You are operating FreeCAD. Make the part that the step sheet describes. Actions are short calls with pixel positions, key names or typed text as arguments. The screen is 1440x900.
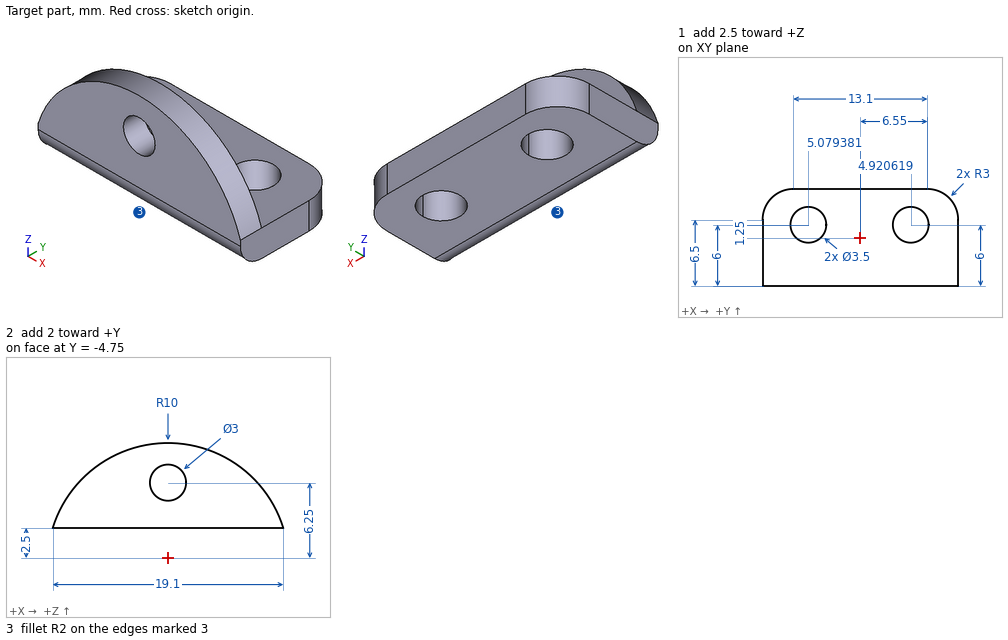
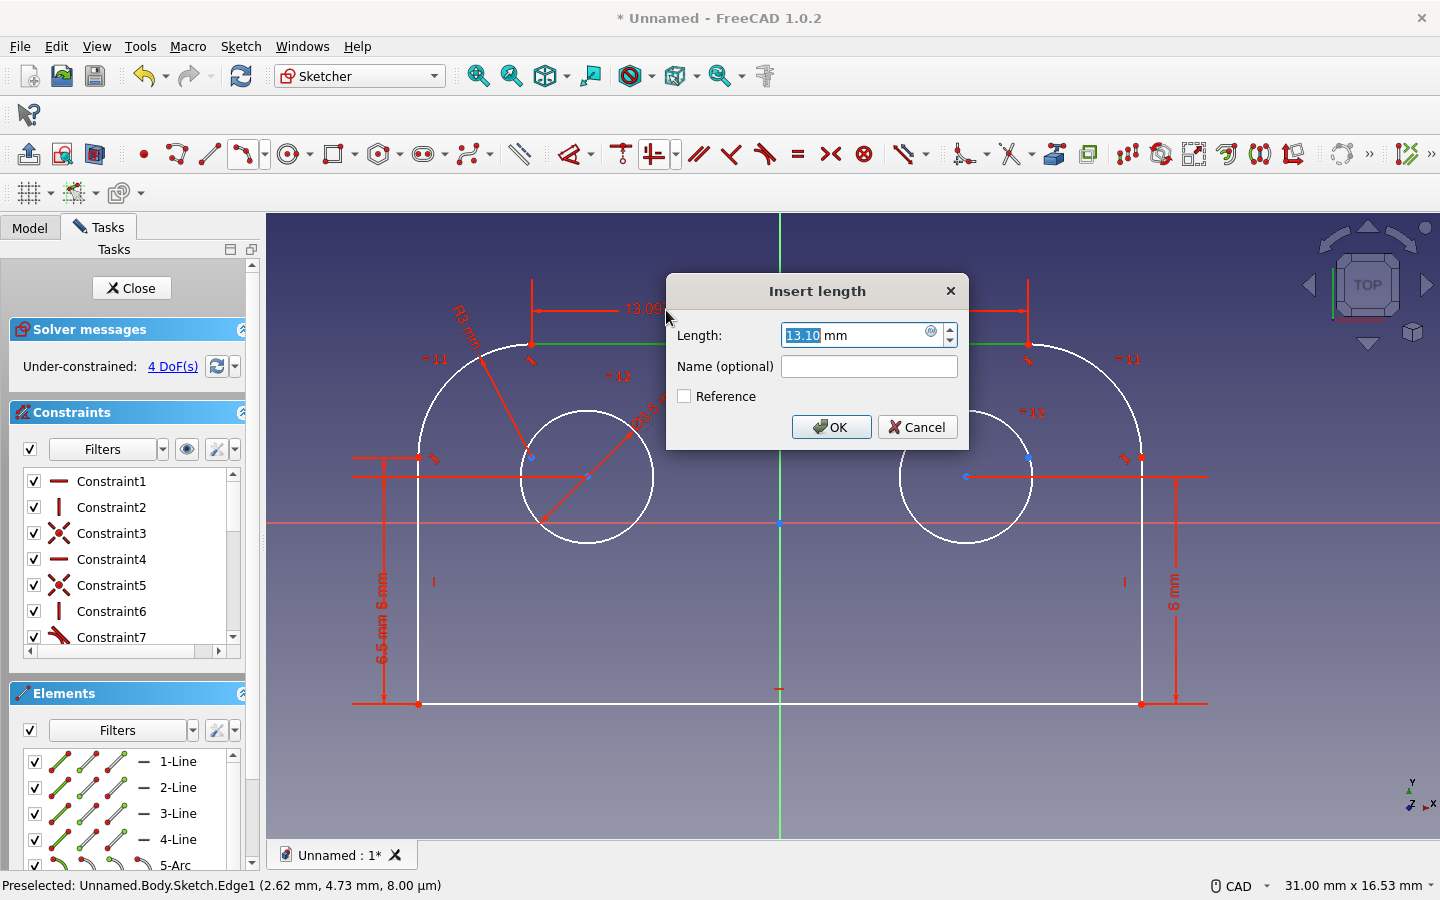
text(13.1)
key(Return)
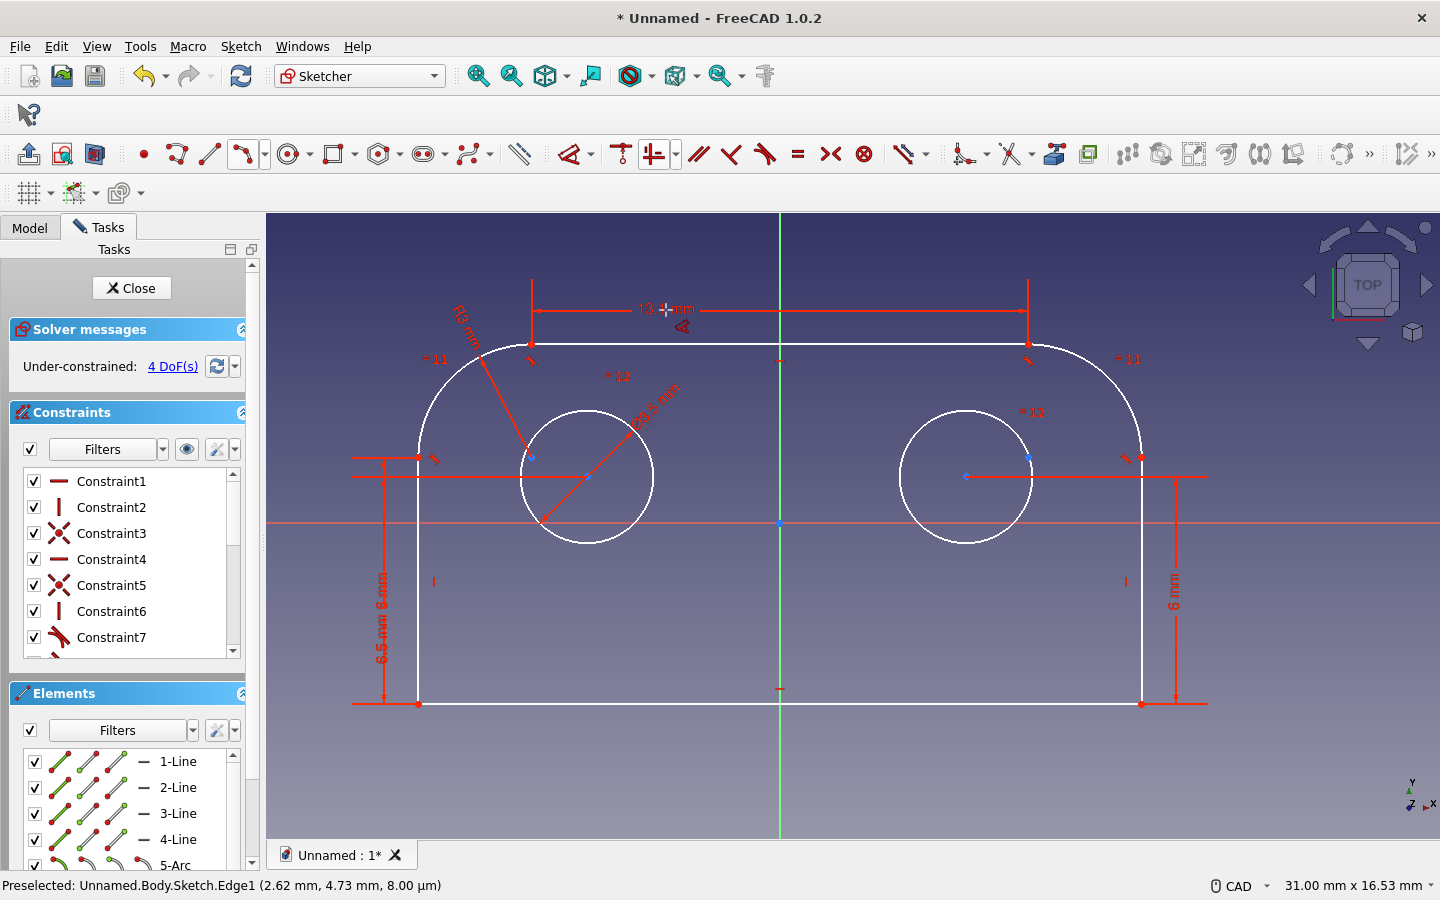
click(587, 477)
click(553, 500)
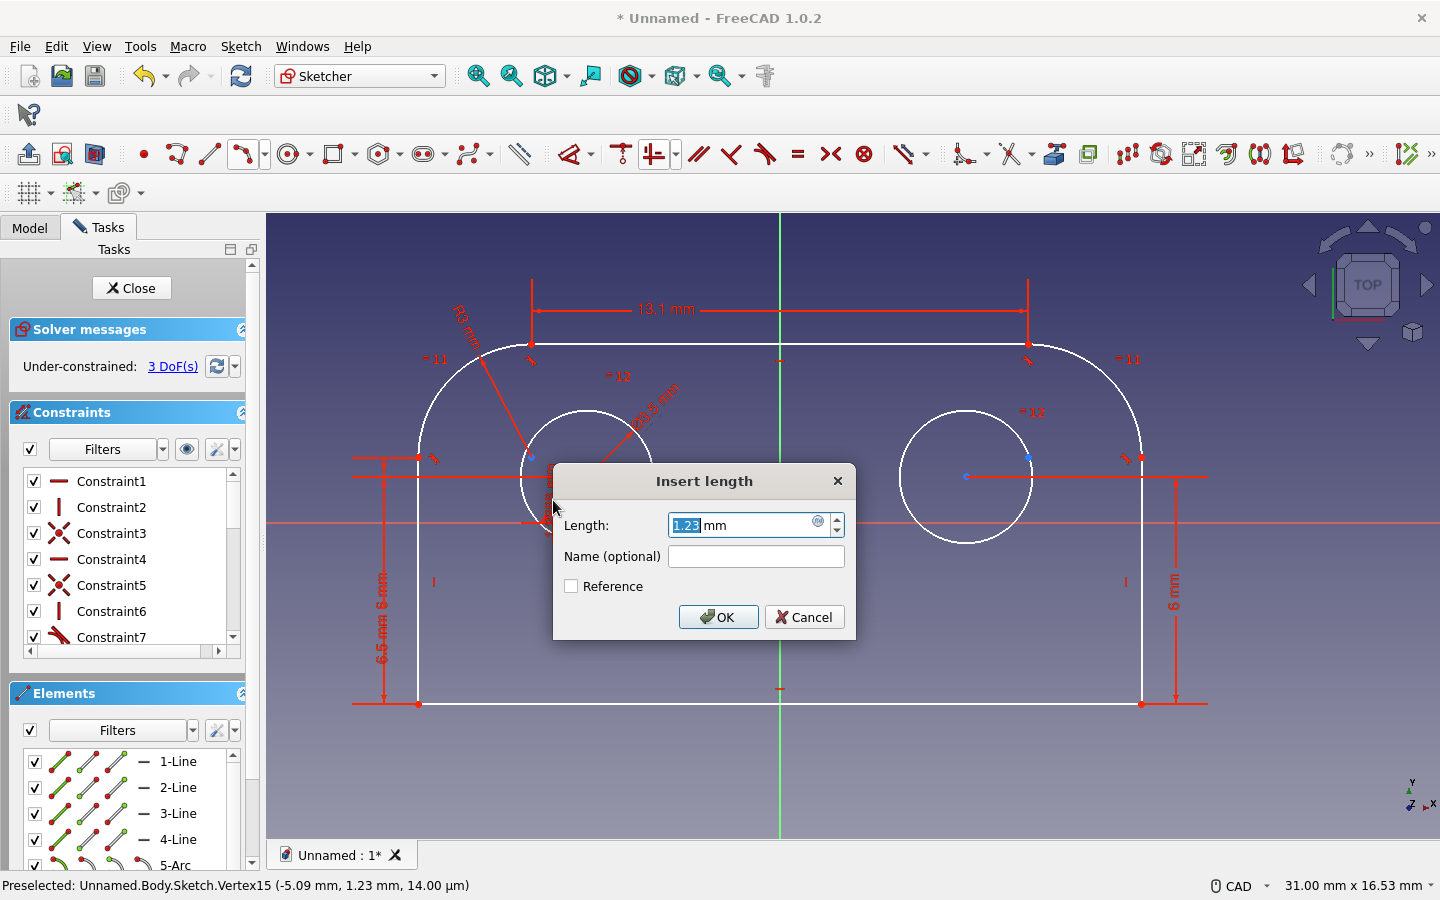
text(1.25)
key(Return)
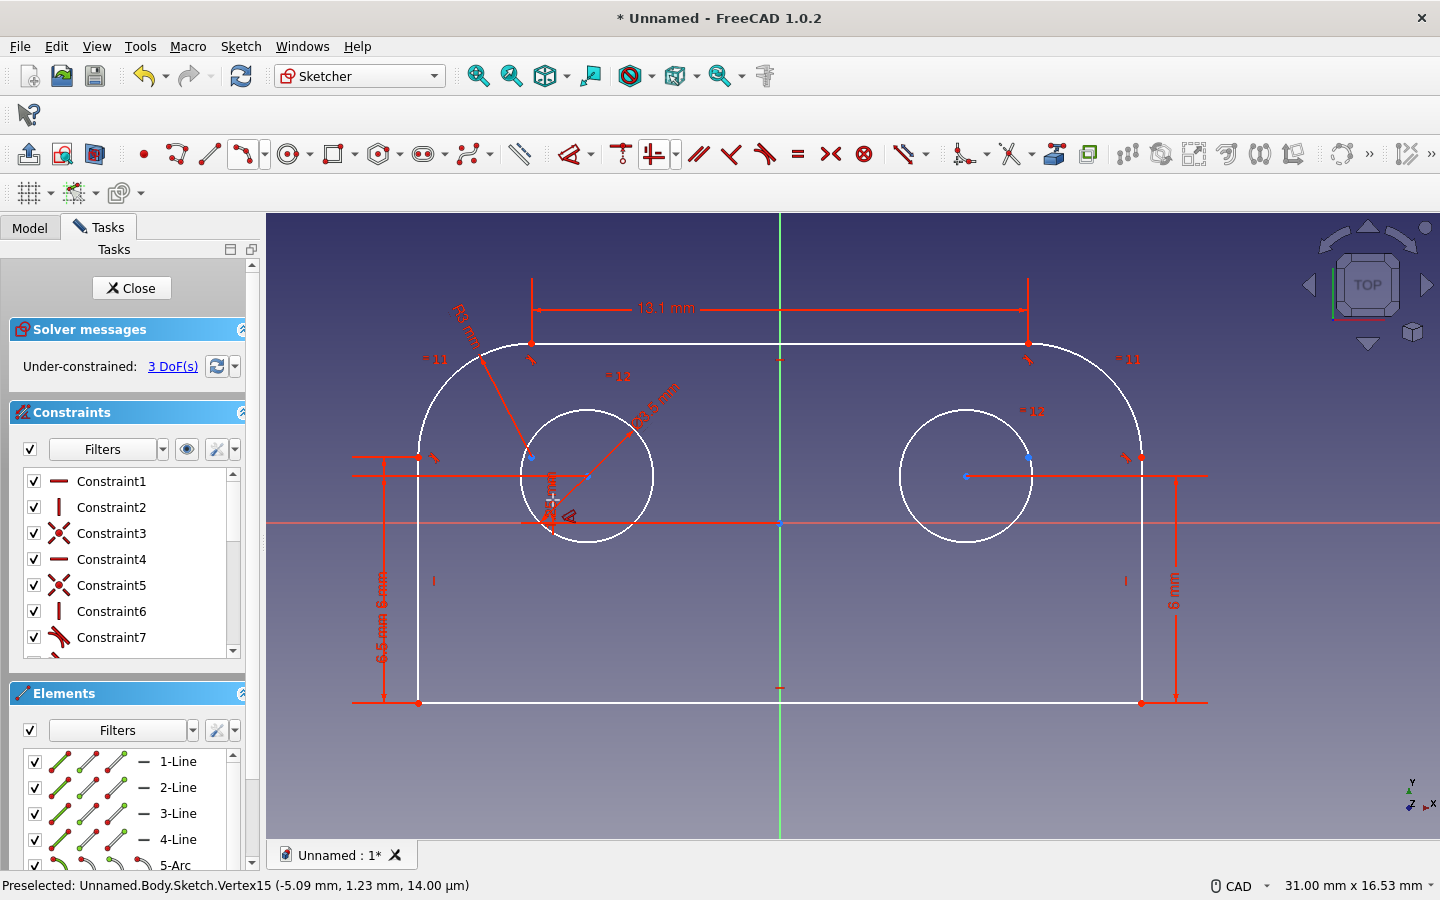
click(1028, 344)
click(904, 310)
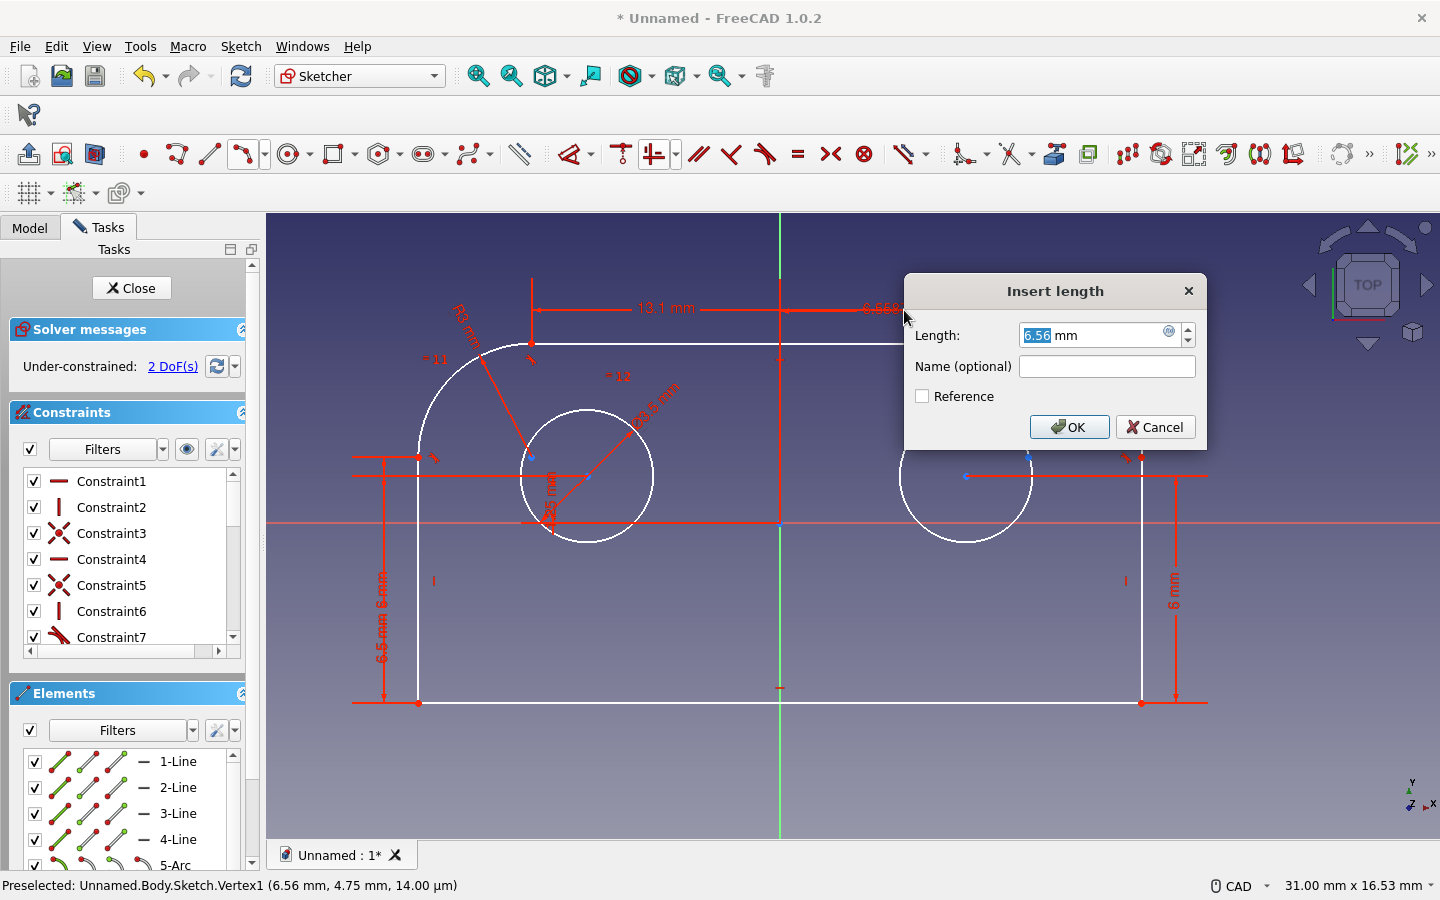
text(6.55)
key(Return)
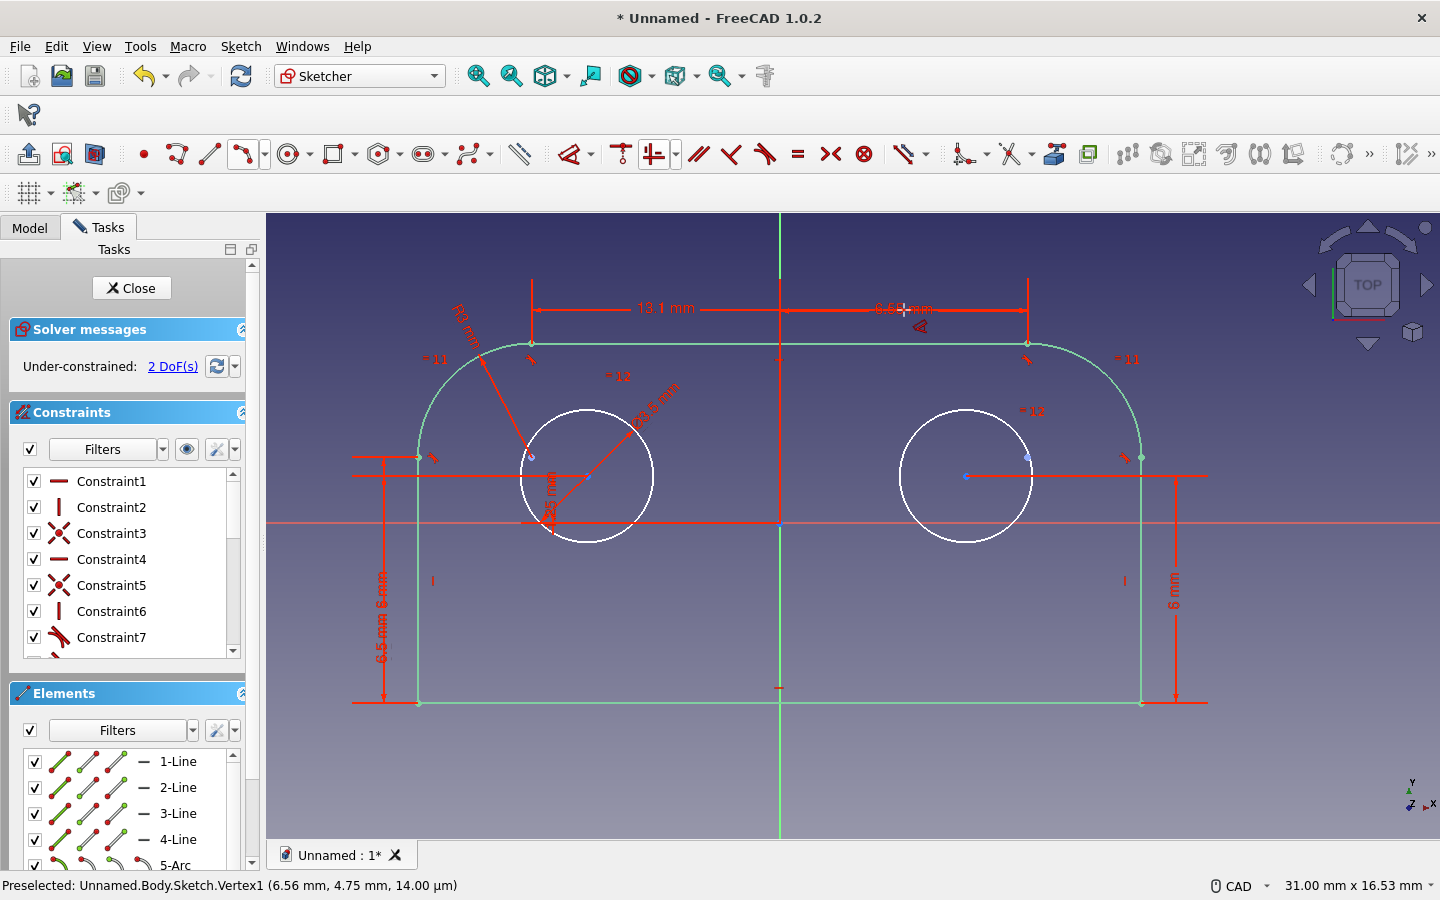
click(587, 476)
click(683, 442)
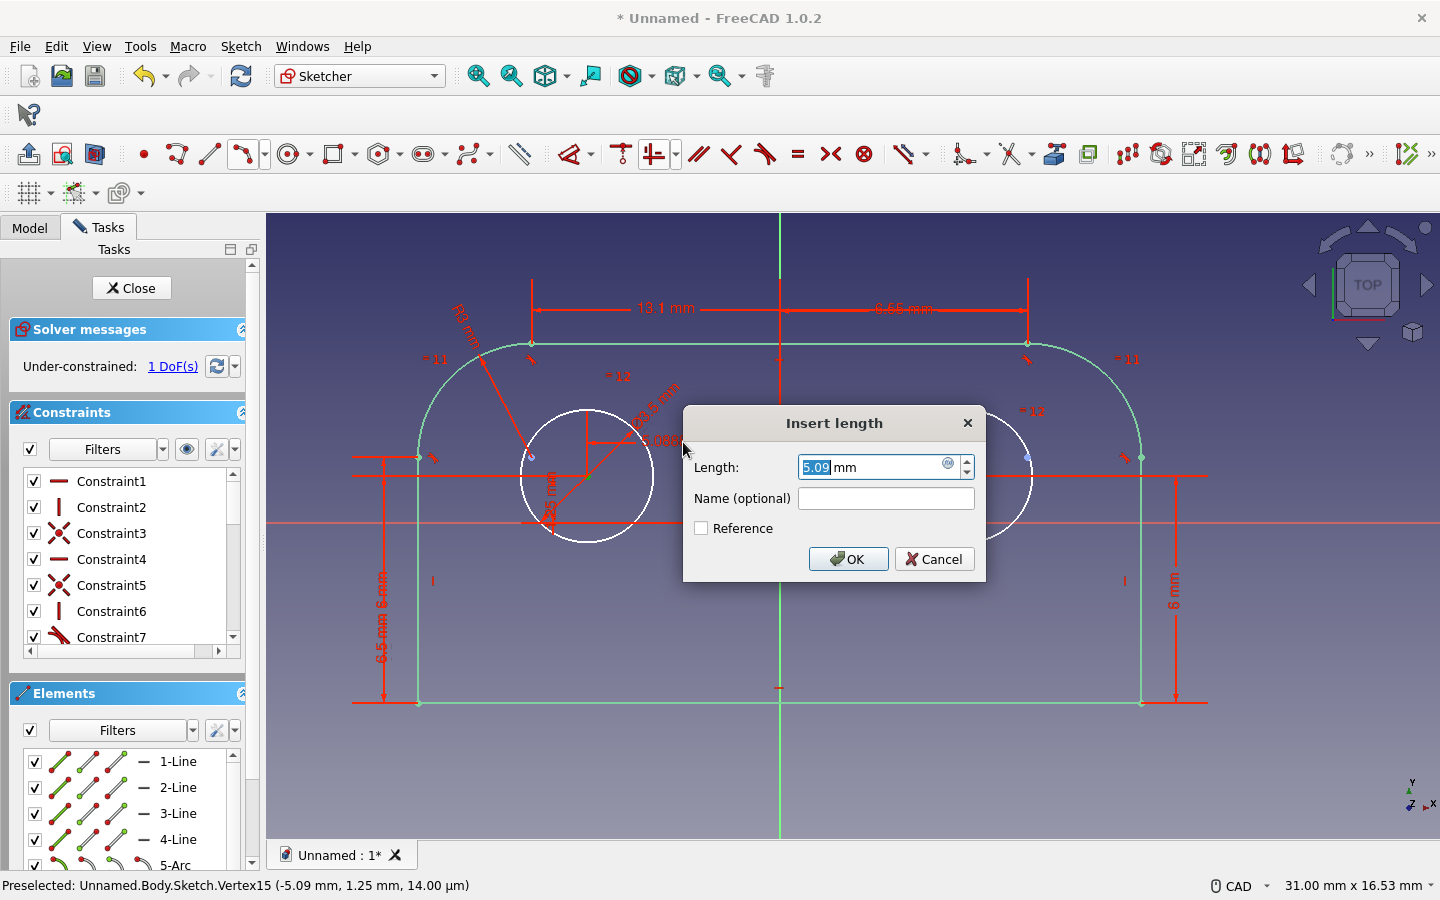
text(5.079381)
key(Return)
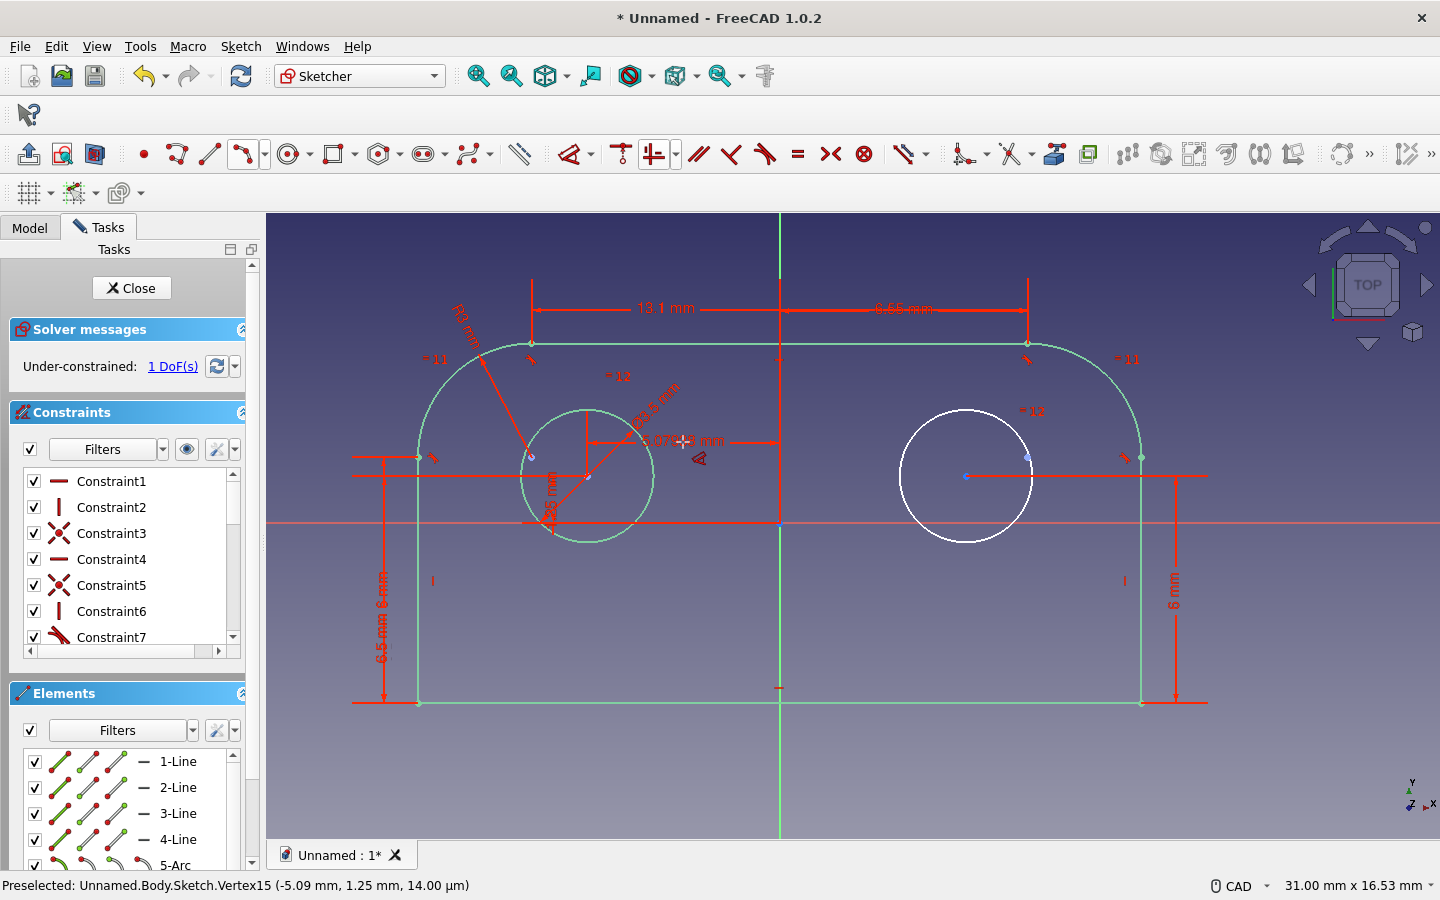
click(966, 476)
click(873, 442)